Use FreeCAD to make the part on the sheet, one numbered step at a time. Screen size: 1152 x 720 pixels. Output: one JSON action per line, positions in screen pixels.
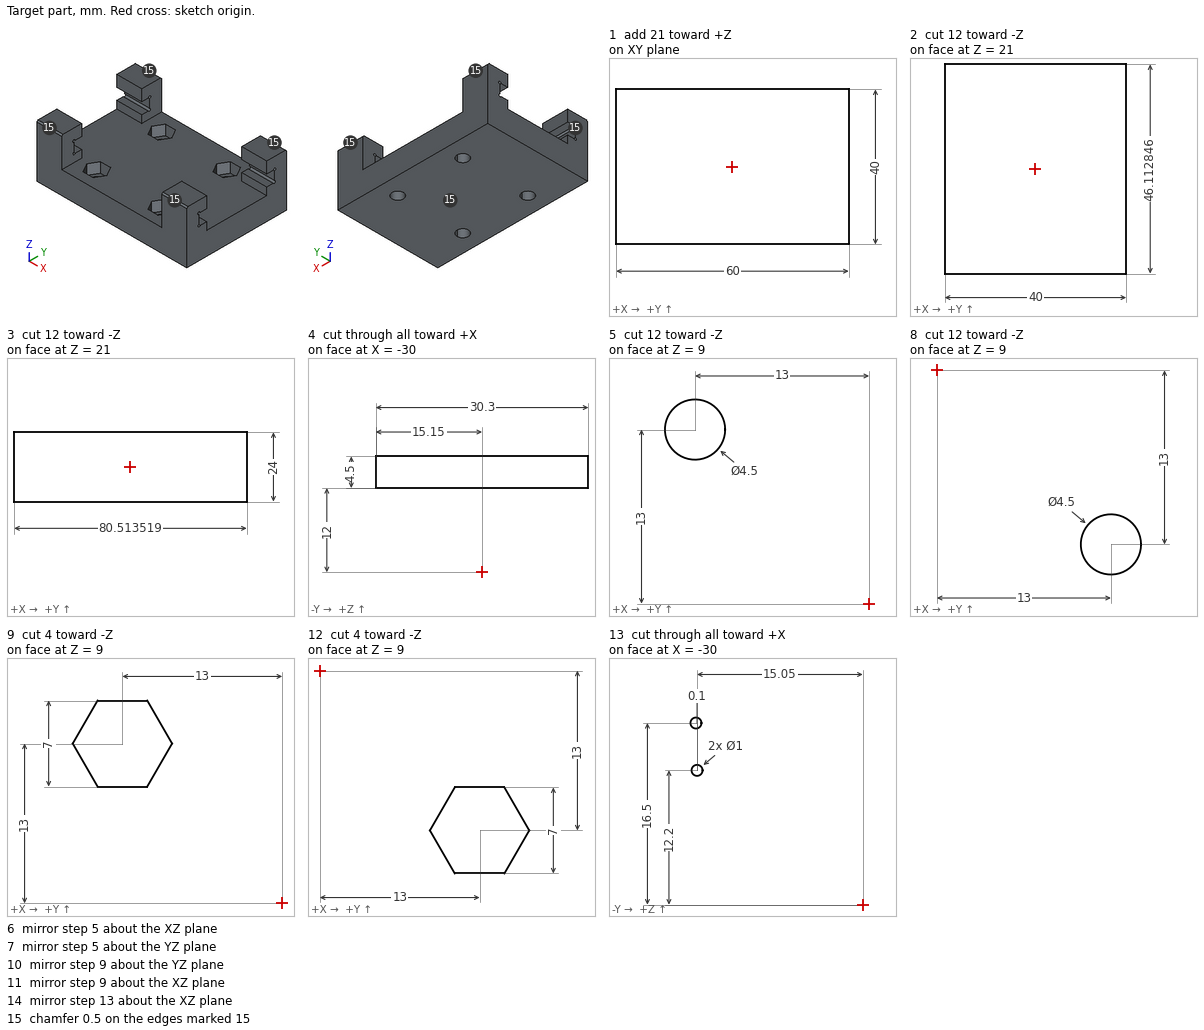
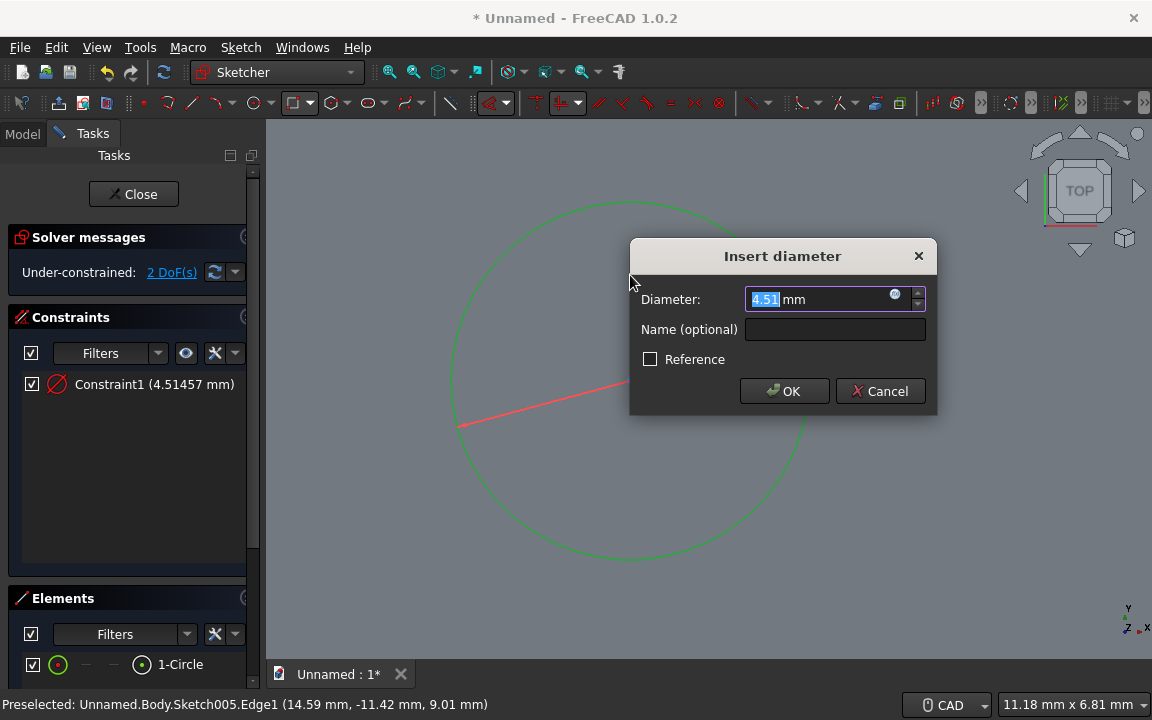
{"action": "type", "text": "4.5"}
{"action": "key", "text": "Return"}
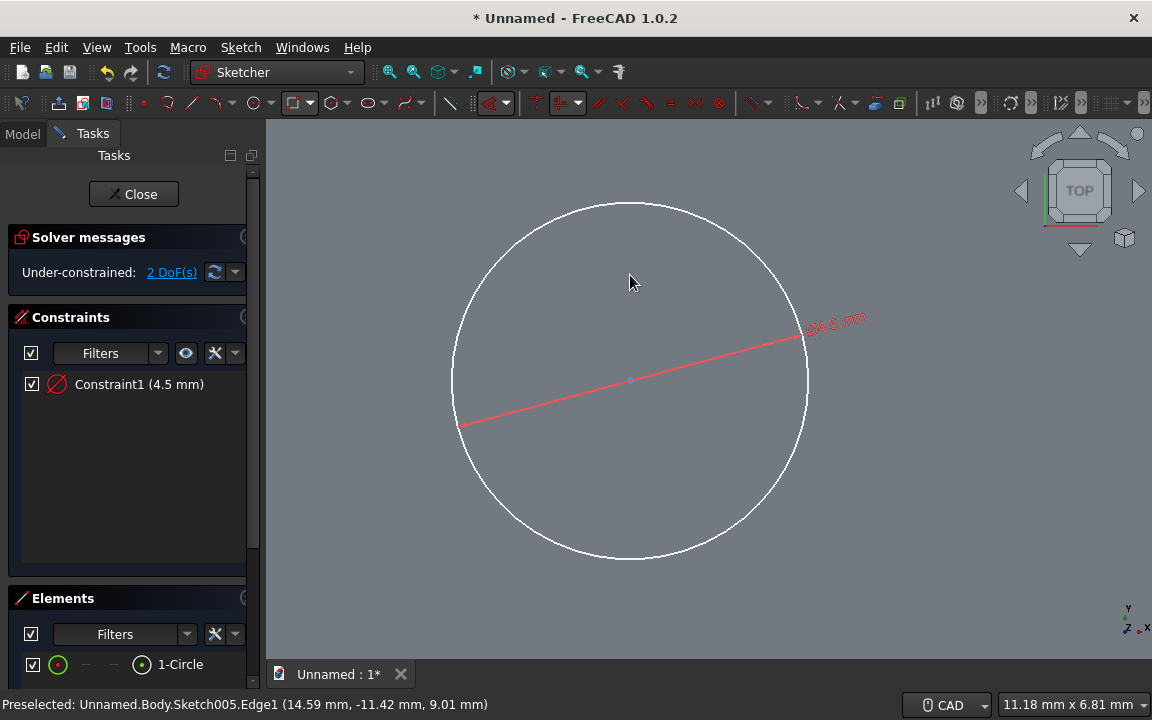
{"action": "left_click", "coordinate": [630, 381]}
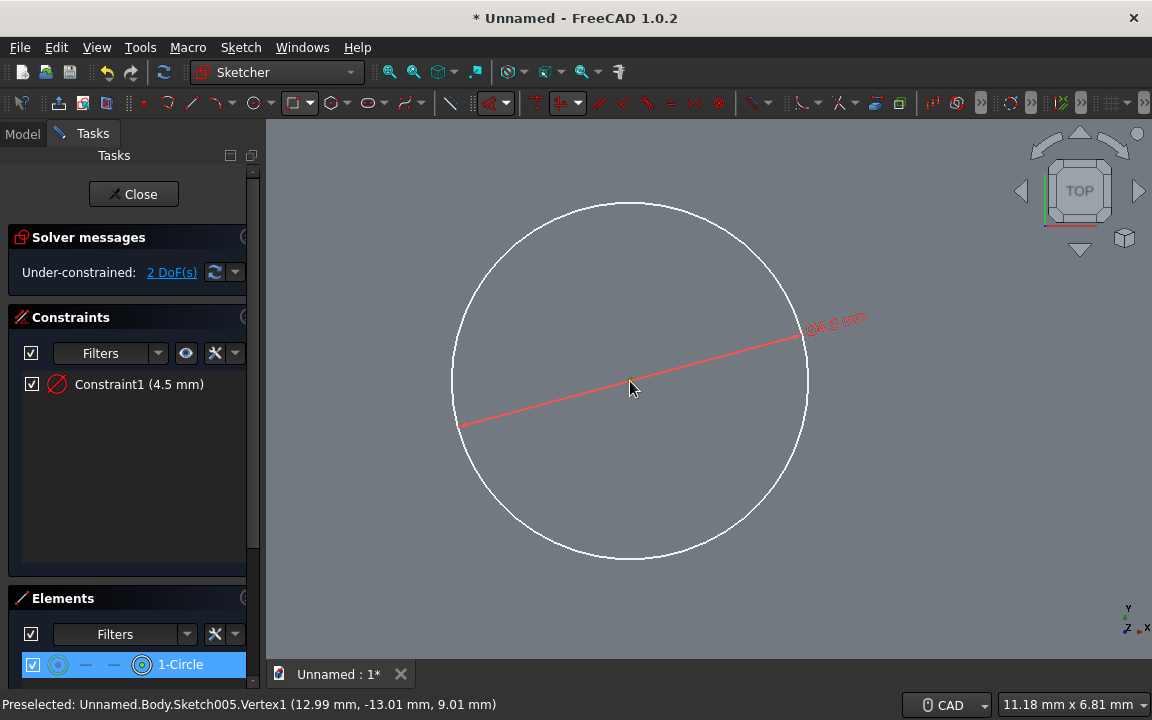
{"action": "left_click", "coordinate": [508, 104]}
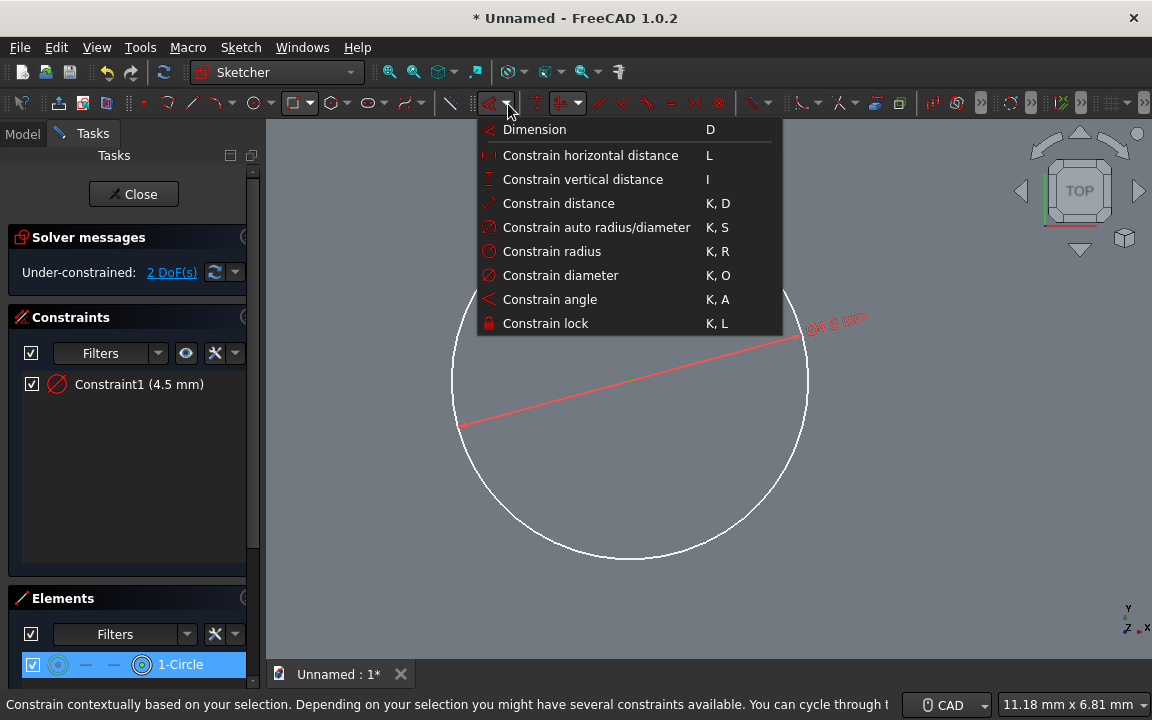
{"action": "left_click", "coordinate": [630, 155]}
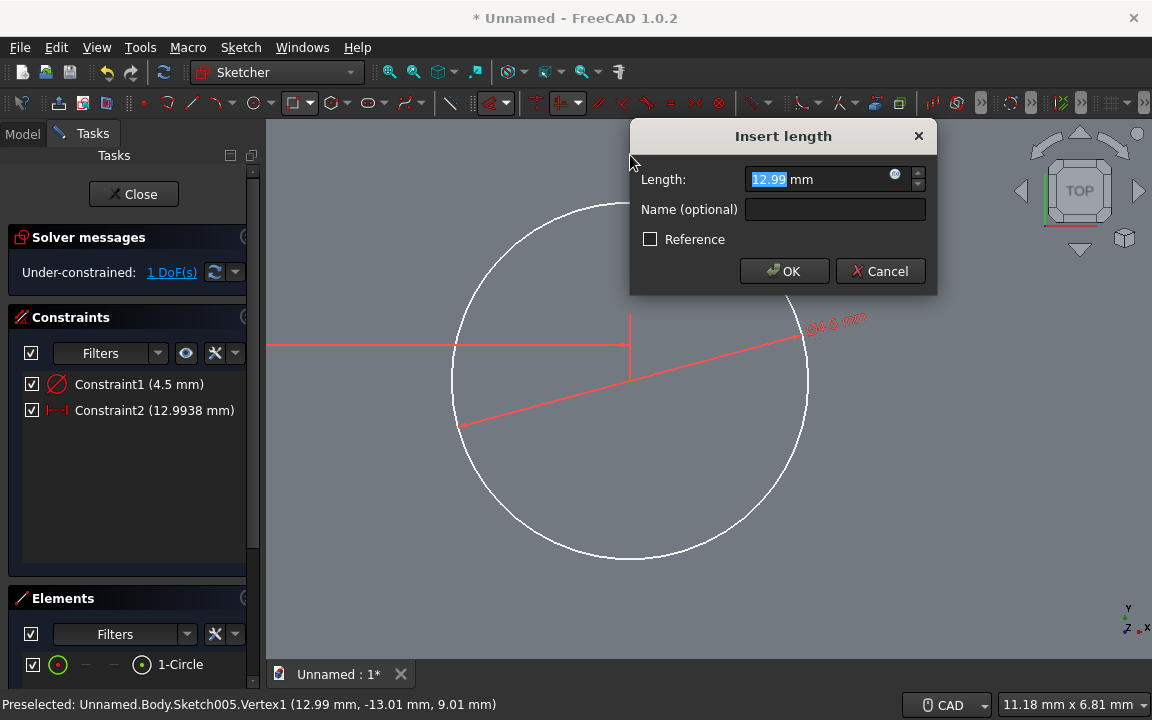
{"action": "type", "text": "13"}
{"action": "key", "text": "Return"}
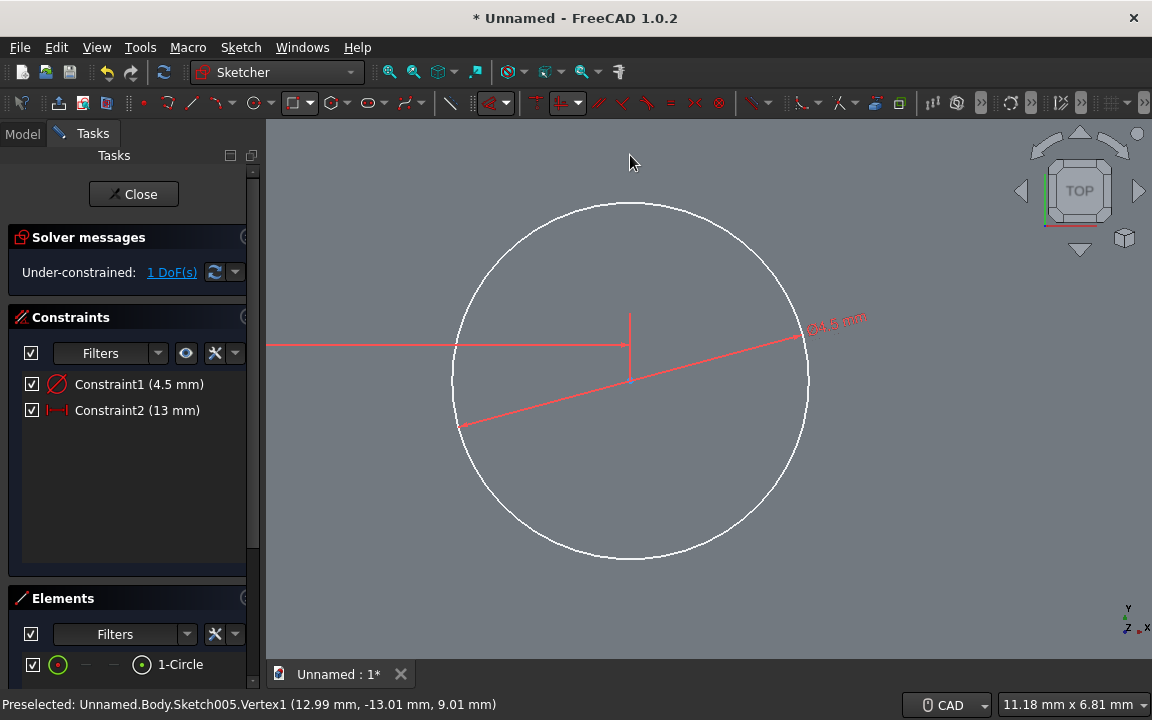
{"action": "left_click", "coordinate": [630, 381]}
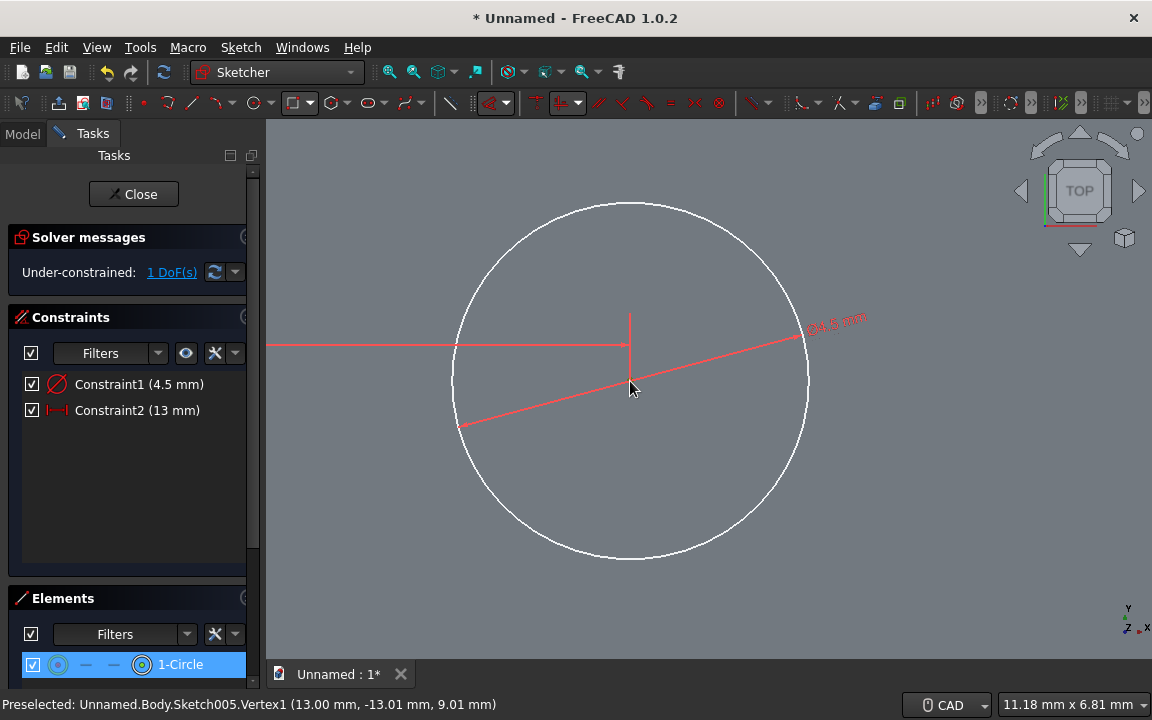
{"action": "left_click", "coordinate": [508, 104]}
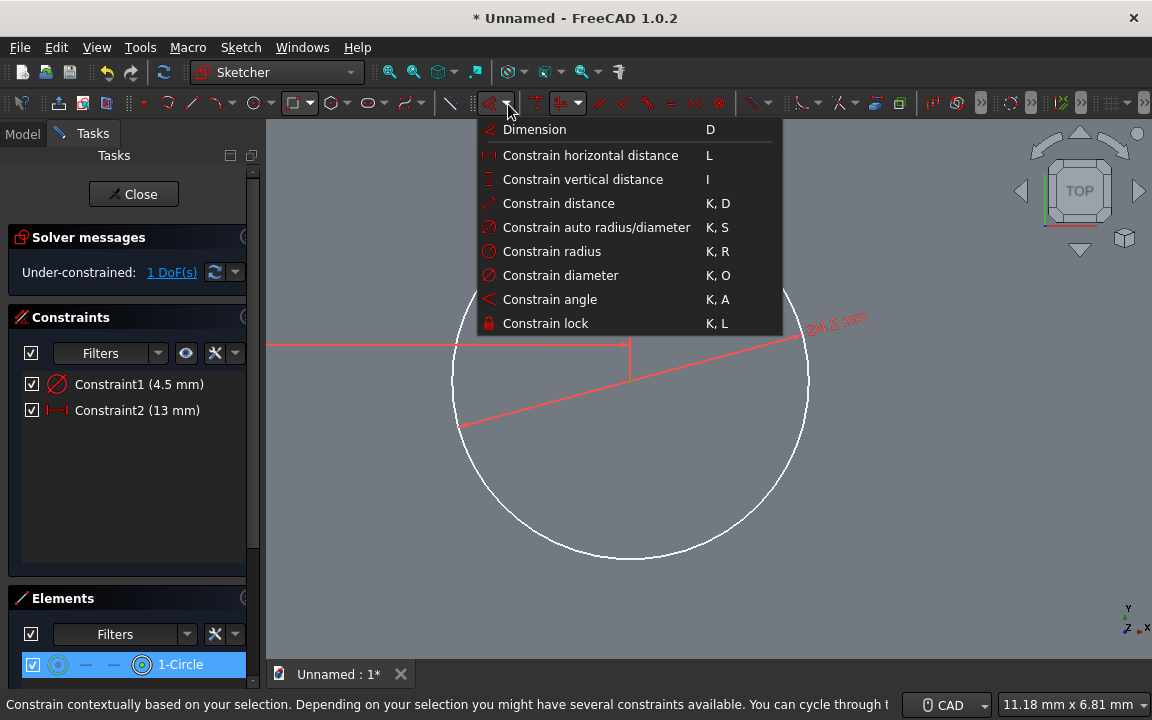
{"action": "left_click", "coordinate": [630, 179]}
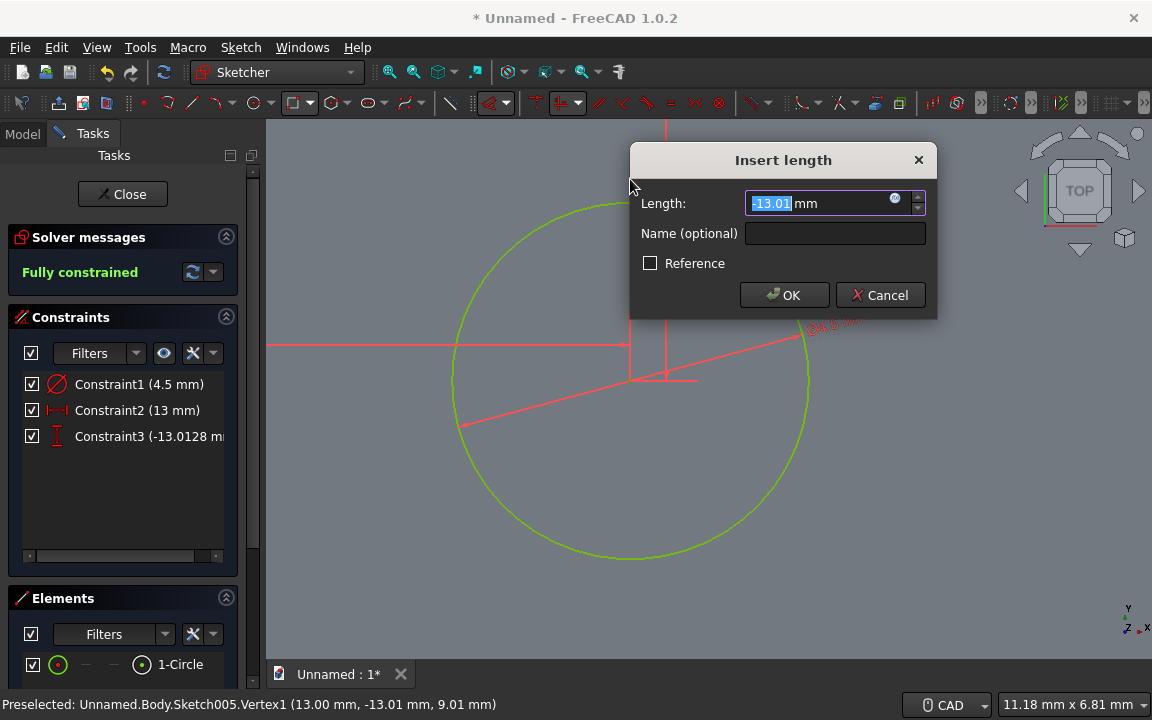
{"action": "type", "text": "-13"}
{"action": "key", "text": "Return"}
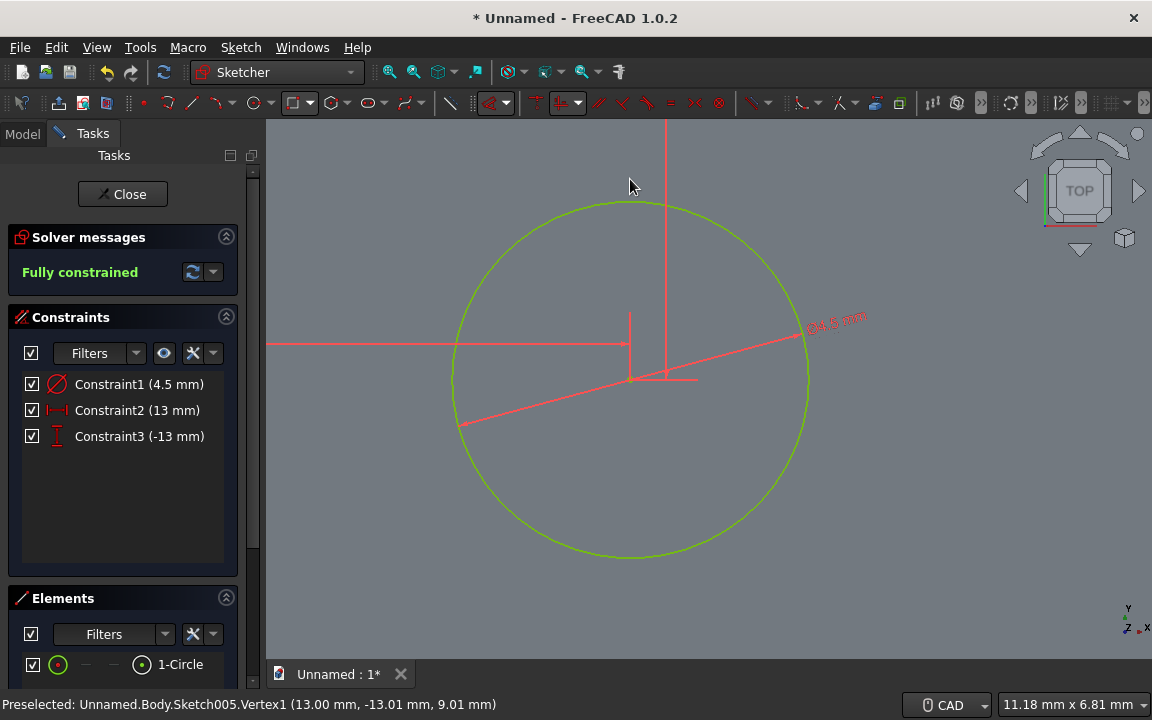
{"action": "left_click", "coordinate": [123, 194]}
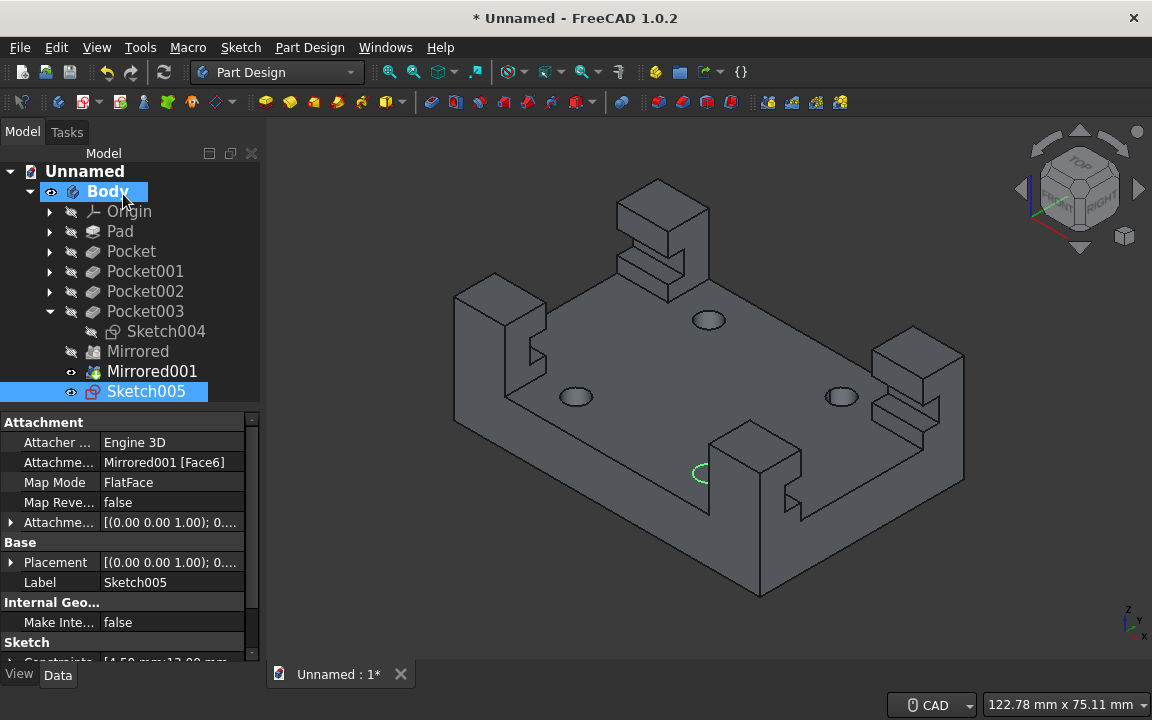
{"action": "left_click", "coordinate": [432, 102]}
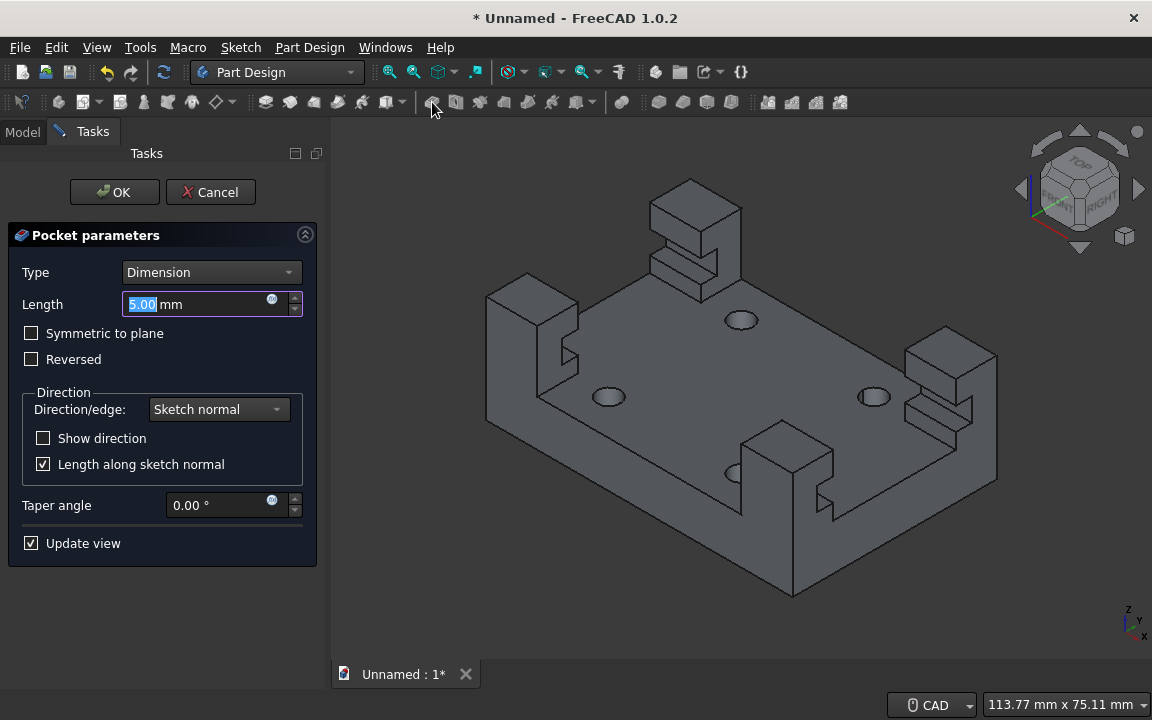
{"action": "type", "text": "12"}
{"action": "key", "text": "Tab"}